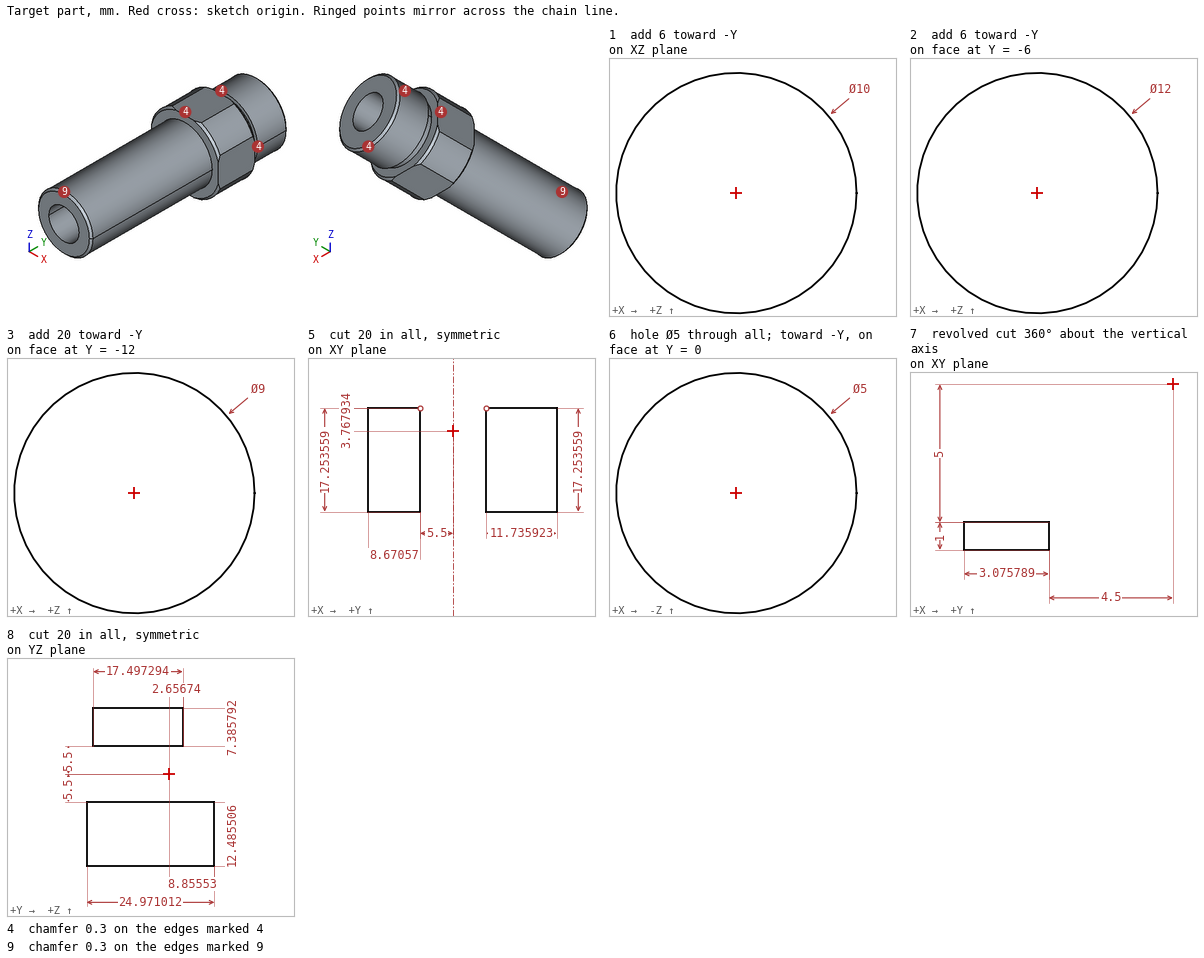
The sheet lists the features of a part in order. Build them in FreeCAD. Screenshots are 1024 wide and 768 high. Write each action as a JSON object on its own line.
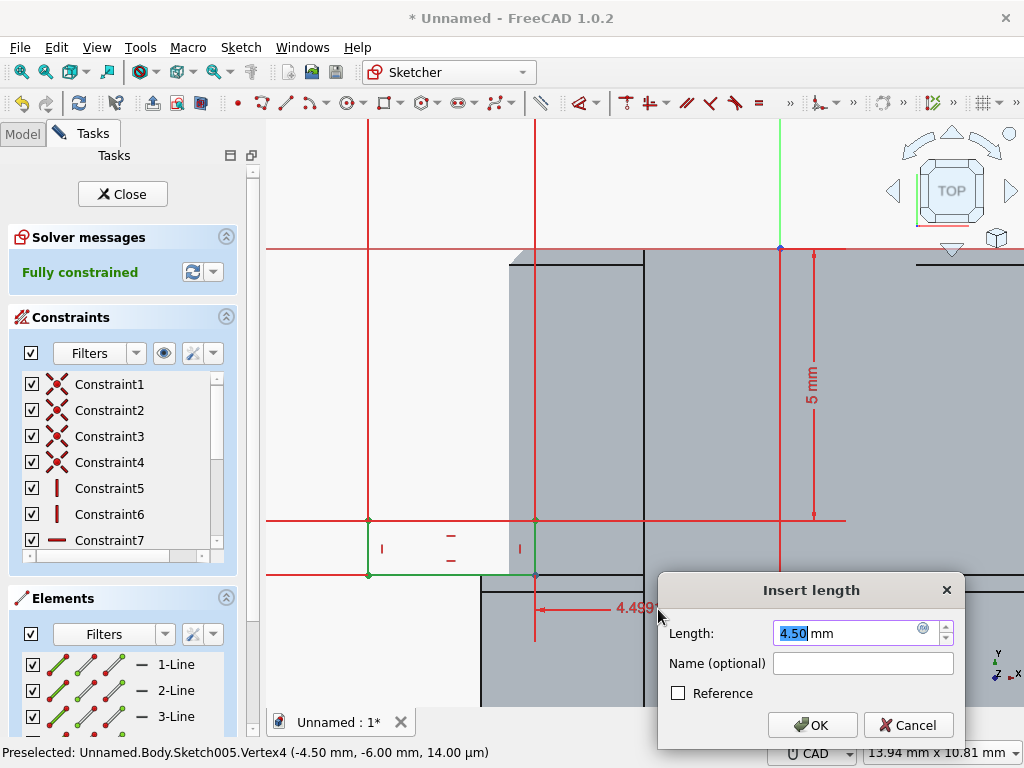
{"action": "type", "text": "4.5"}
{"action": "key", "text": "Return"}
{"action": "key", "text": "Escape"}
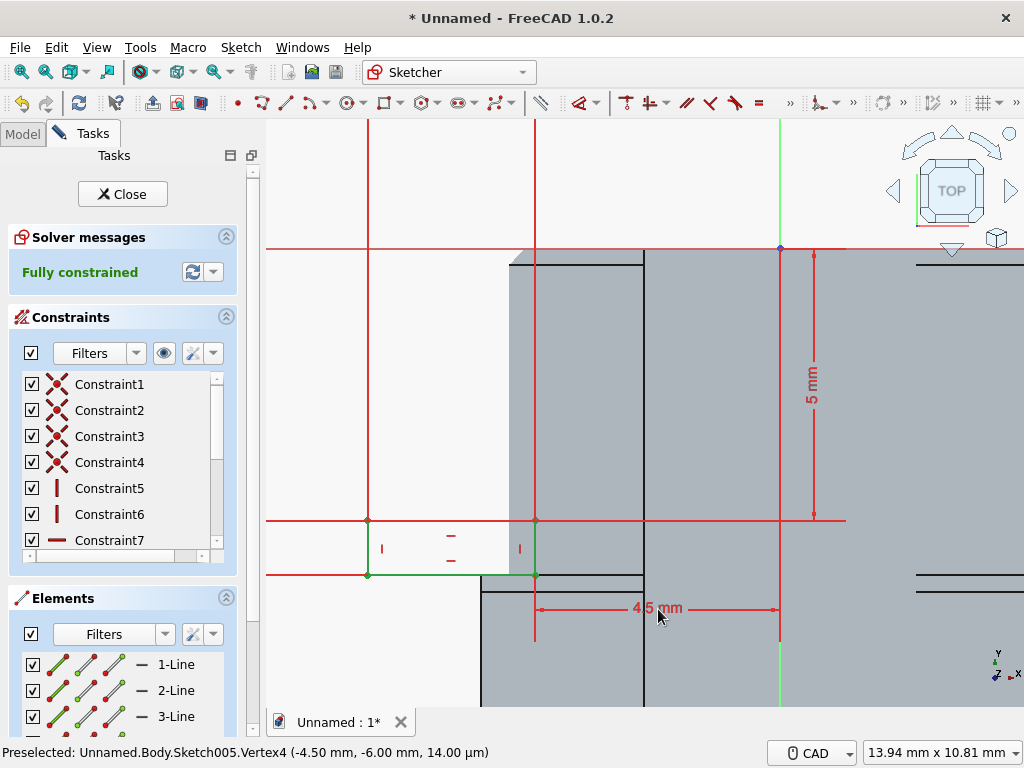
{"action": "left_click", "coordinate": [123, 194]}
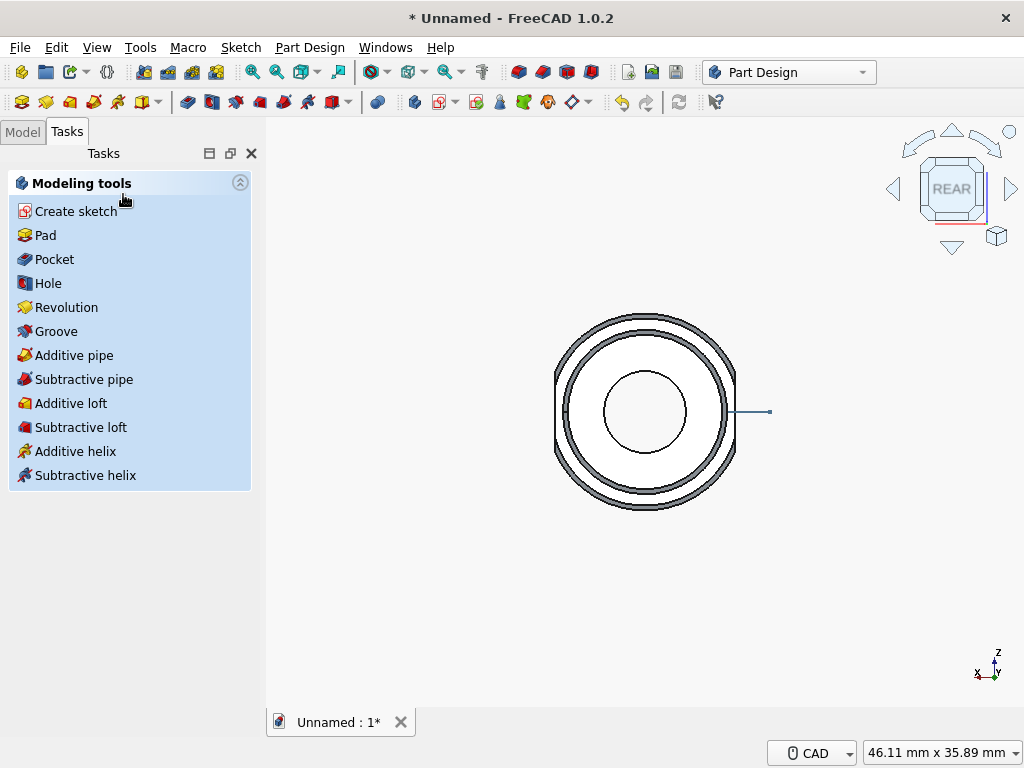
{"action": "left_click", "coordinate": [236, 102]}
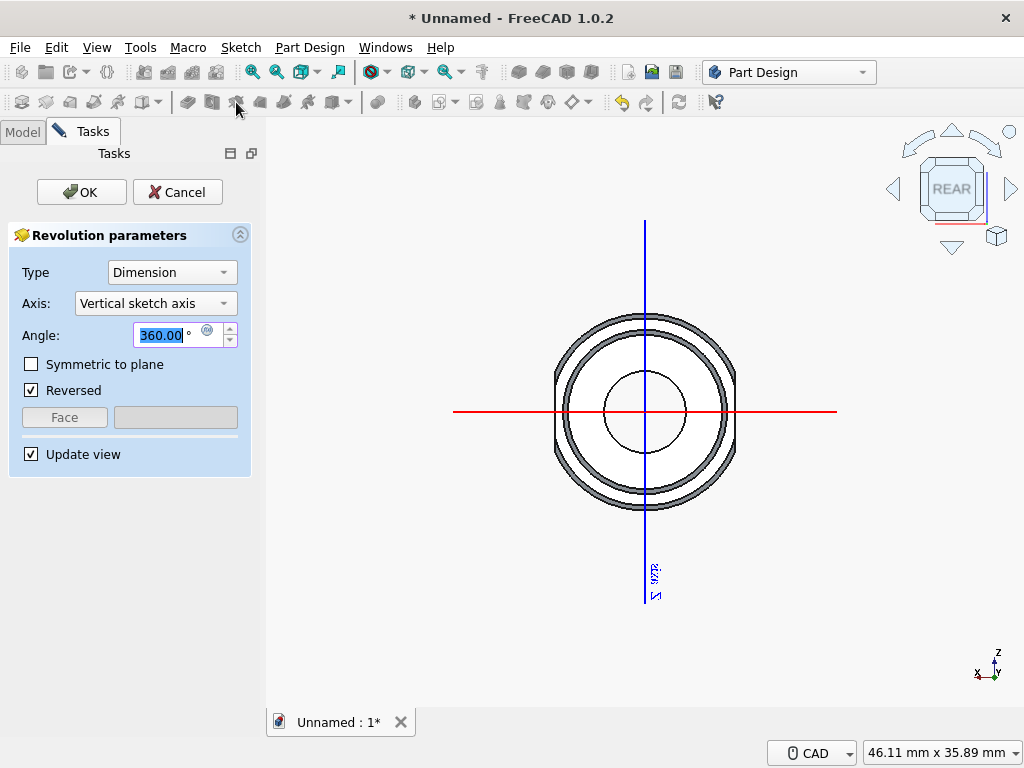
{"action": "left_click", "coordinate": [82, 192]}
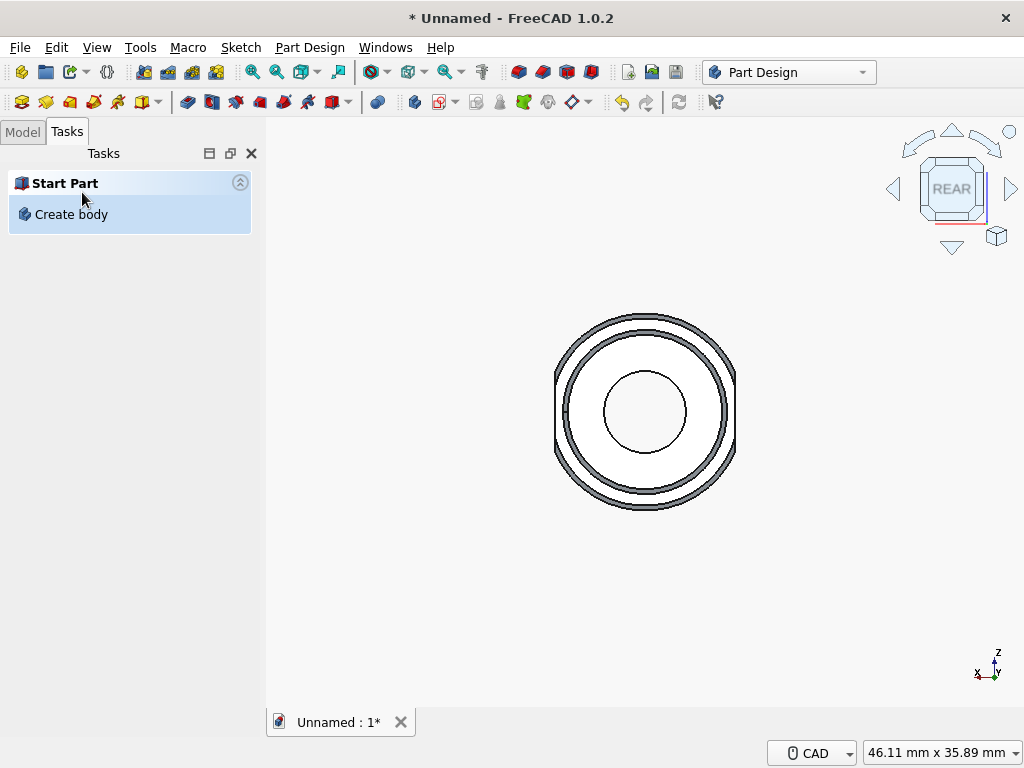
{"action": "key", "text": "v f"}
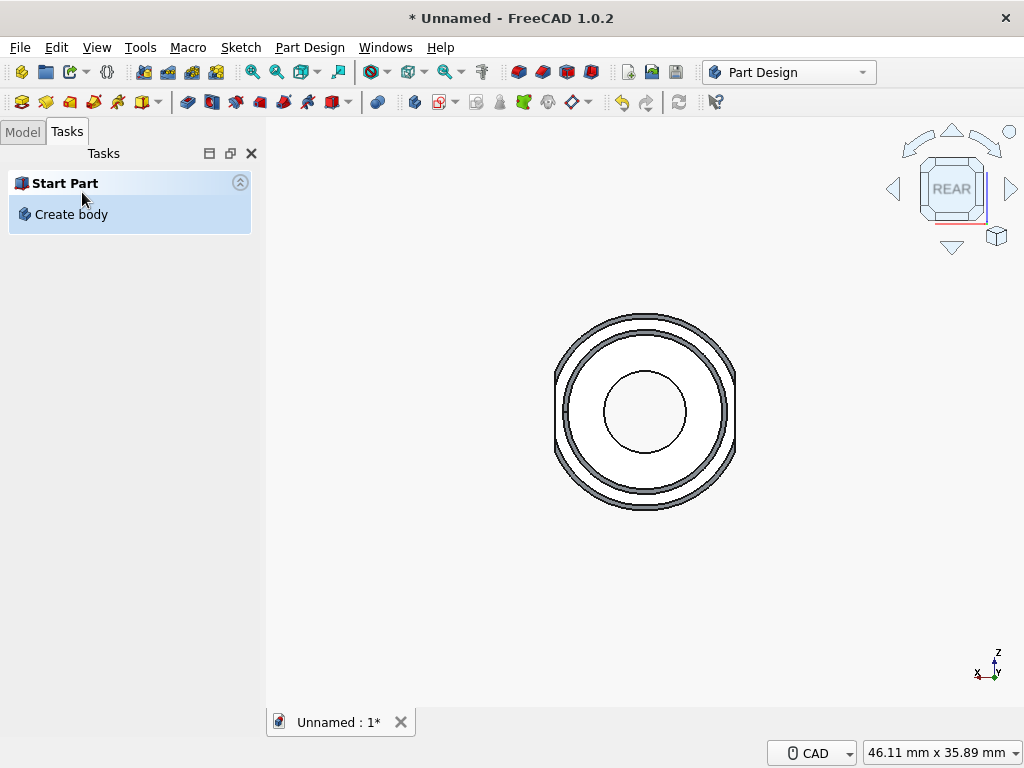
{"action": "left_click", "coordinate": [440, 102]}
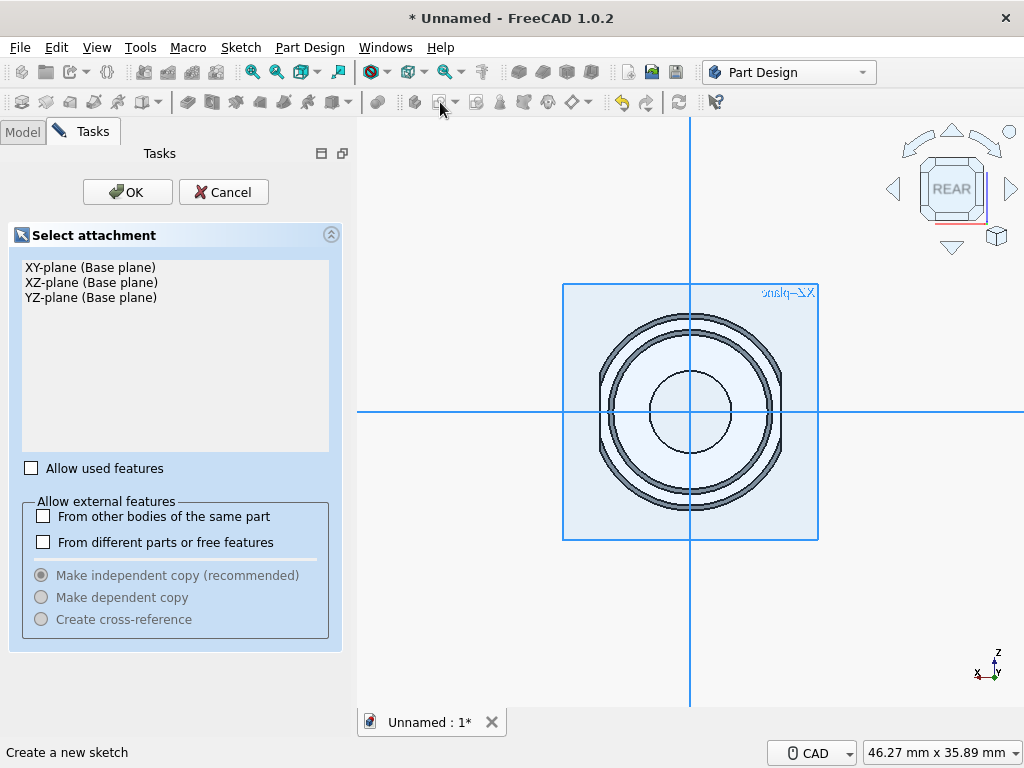
{"action": "left_click", "coordinate": [82, 298]}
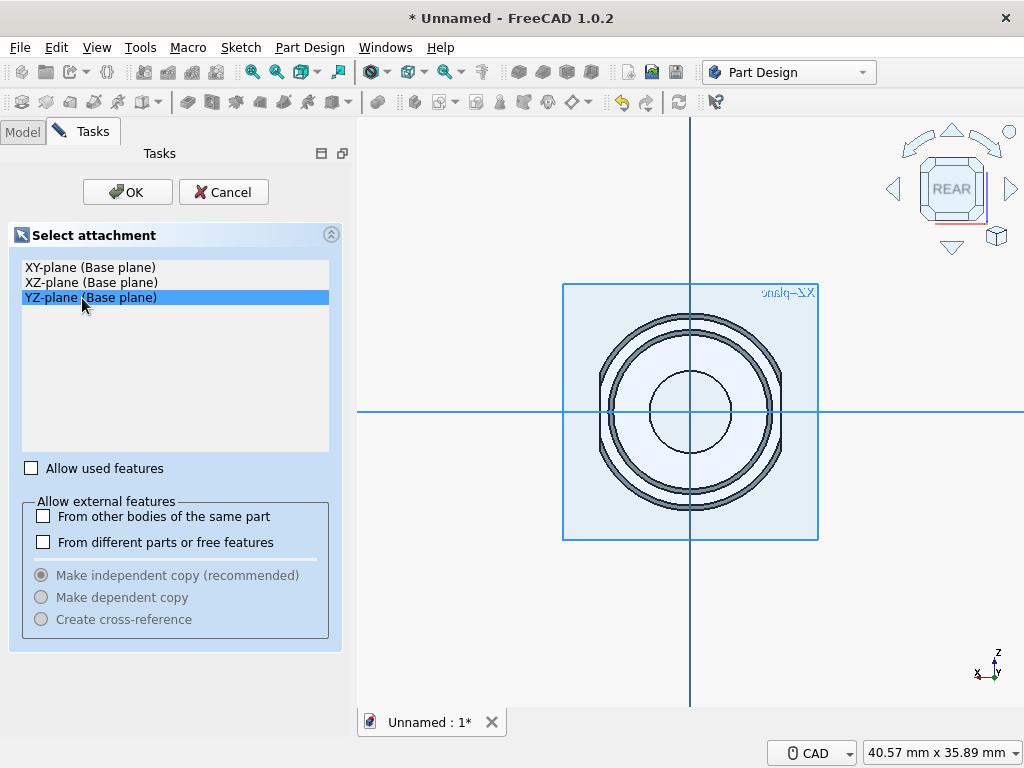
{"action": "left_click", "coordinate": [128, 192]}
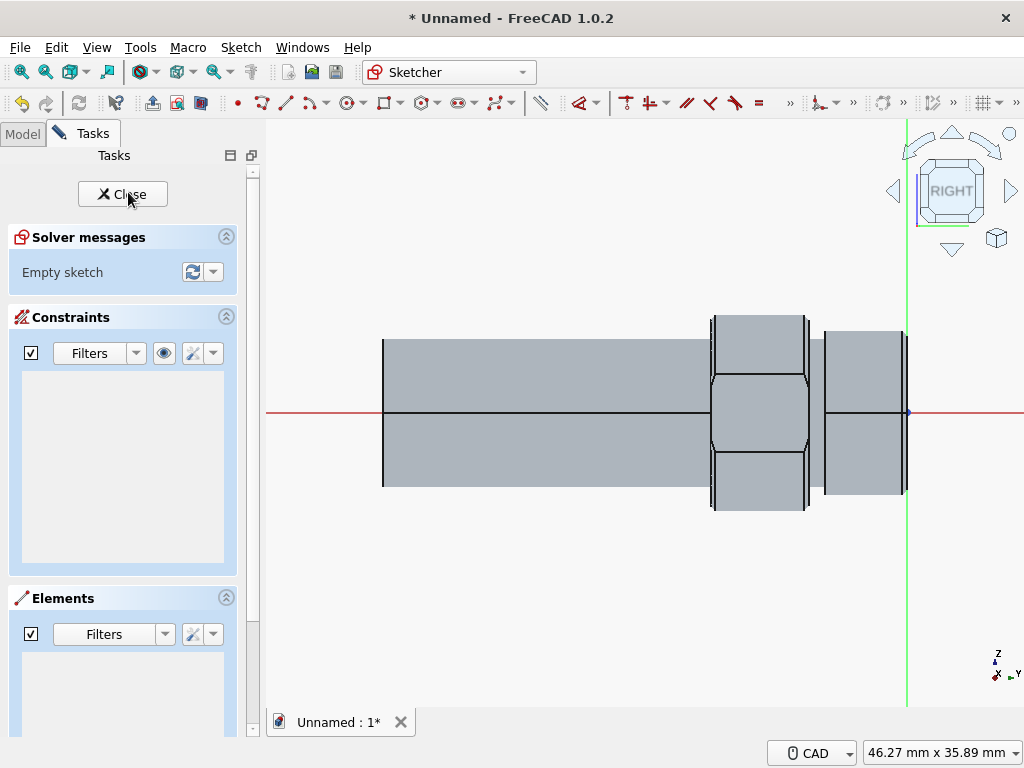
{"action": "left_click", "coordinate": [202, 104]}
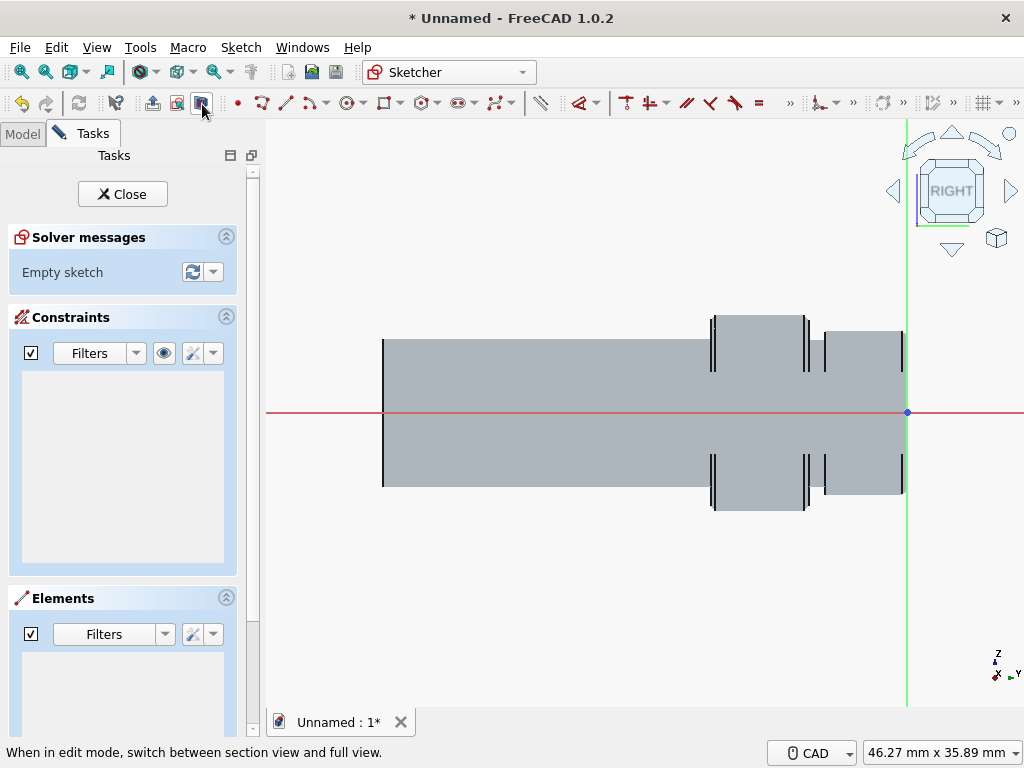
{"action": "scroll", "coordinate": [294, 328], "scroll_direction": "down", "scroll_amount": 2}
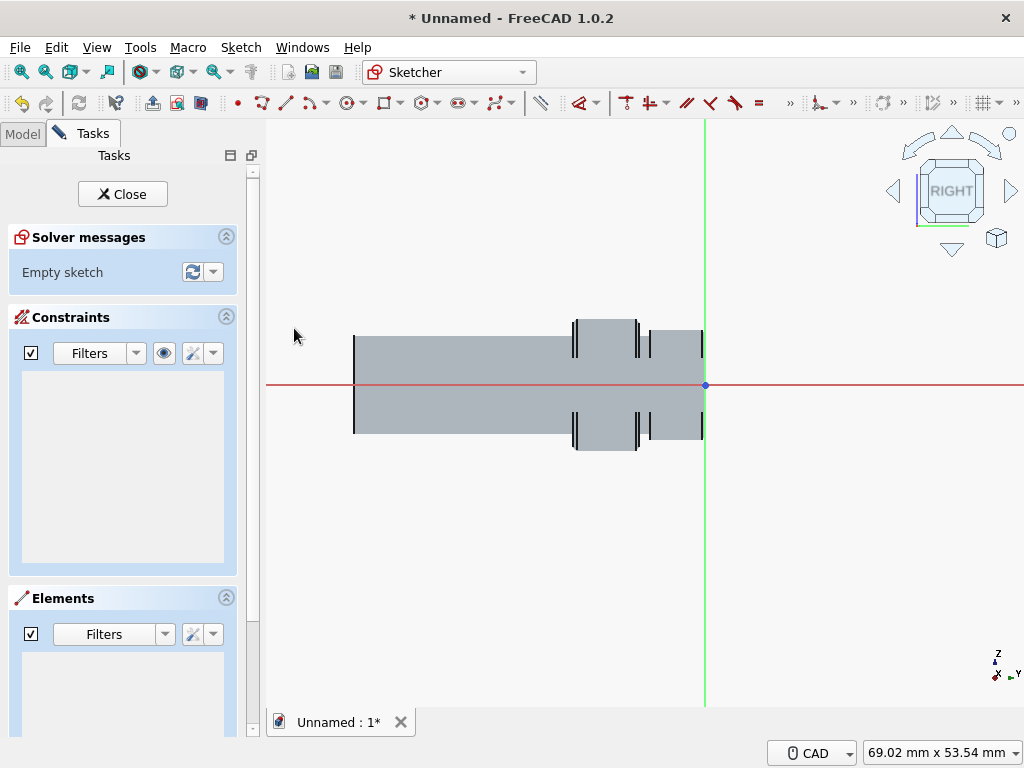
{"action": "key", "text": "g r"}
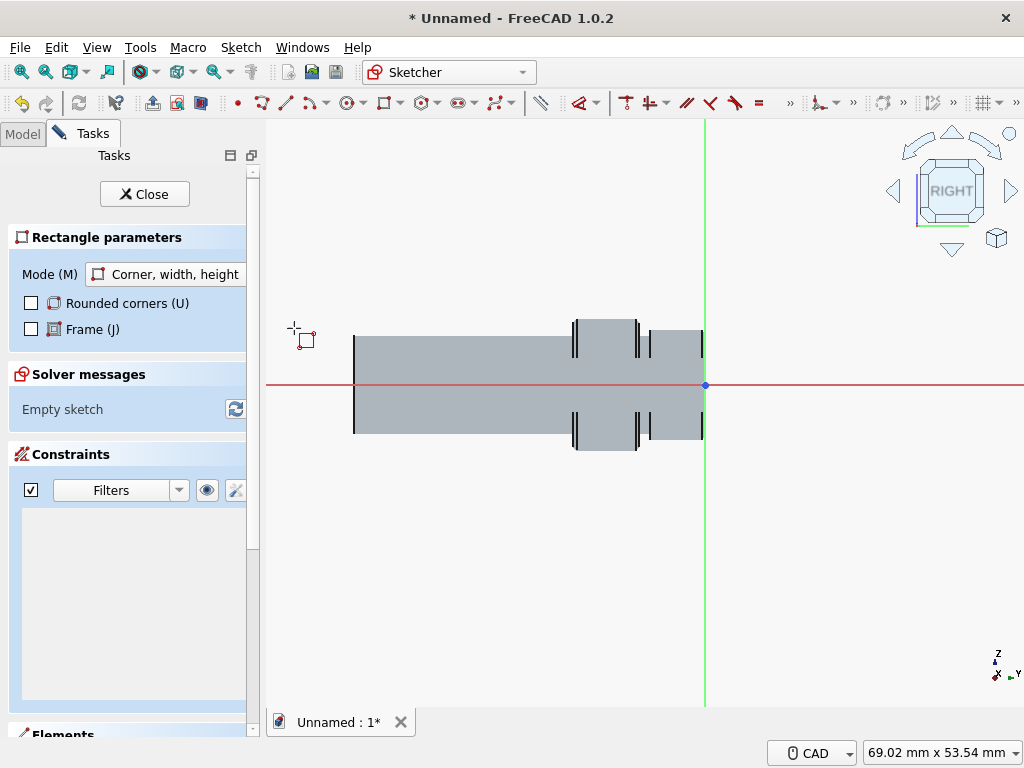
{"action": "left_click", "coordinate": [542, 244]}
{"action": "mouse_move", "coordinate": [734, 325]}